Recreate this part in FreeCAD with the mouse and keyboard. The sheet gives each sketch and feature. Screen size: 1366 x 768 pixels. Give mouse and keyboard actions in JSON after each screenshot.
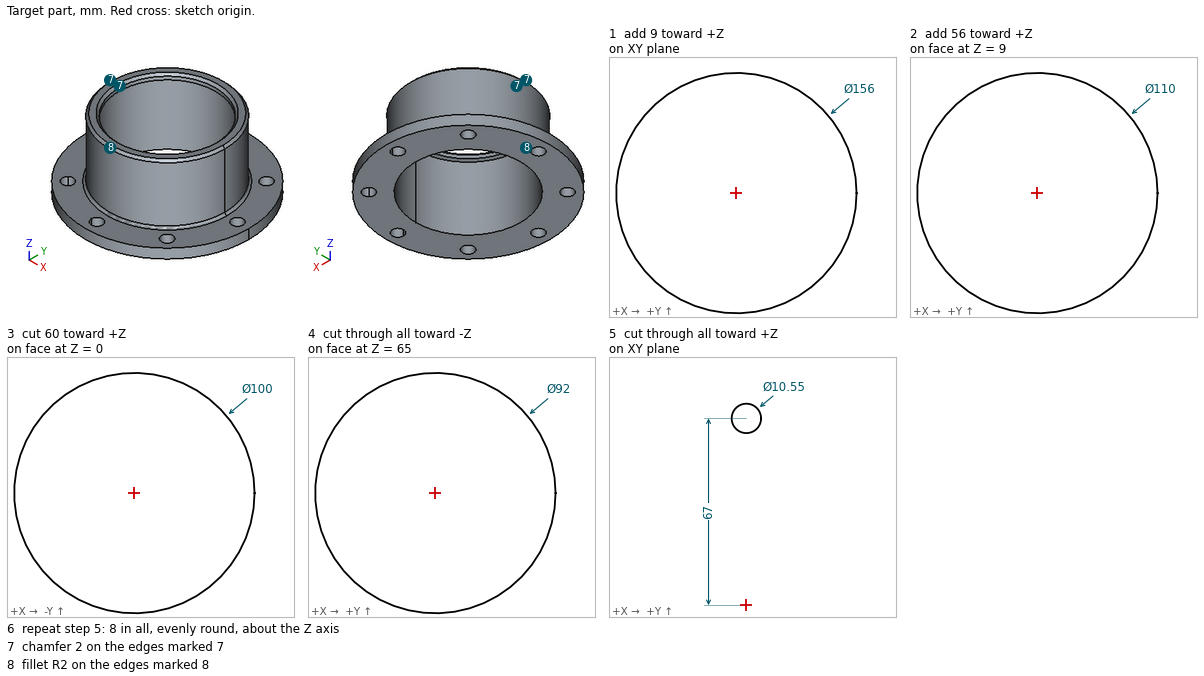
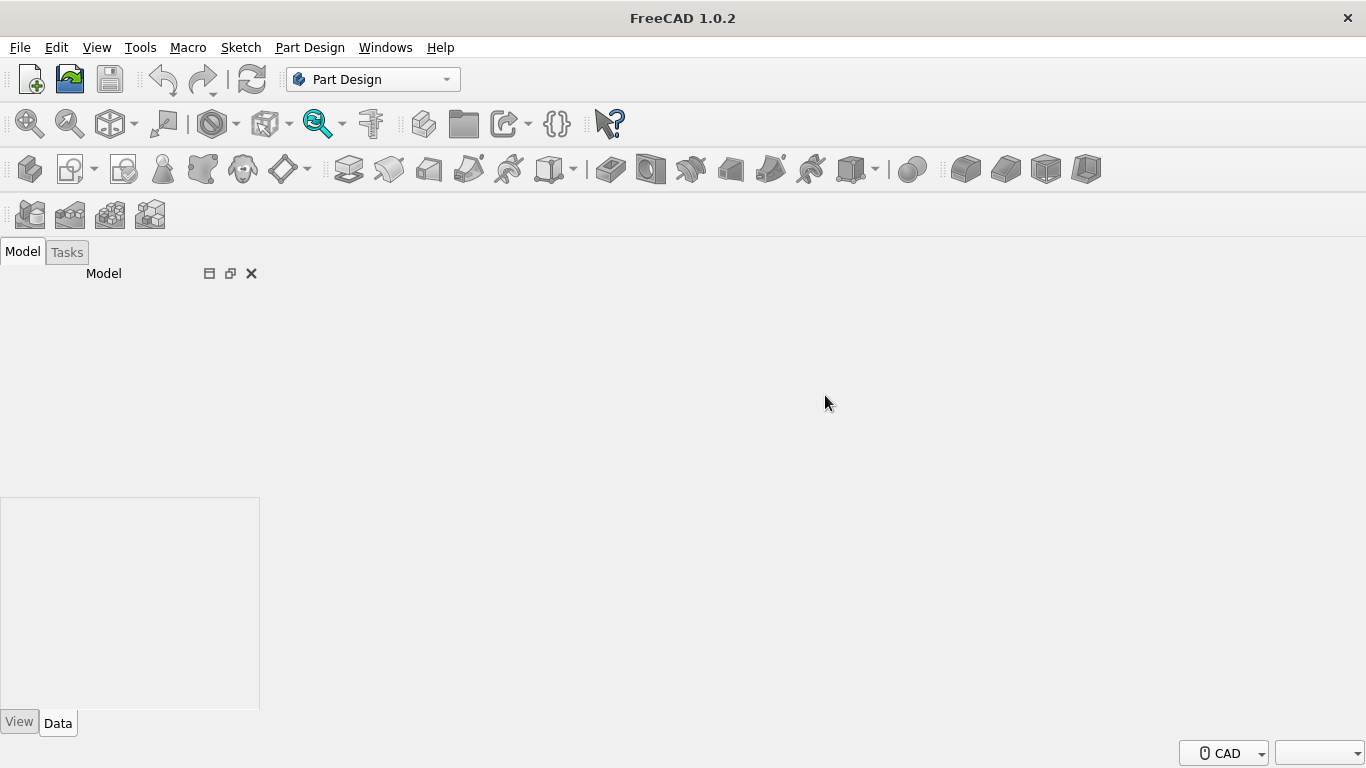
{"action": "key", "text": "ctrl+n"}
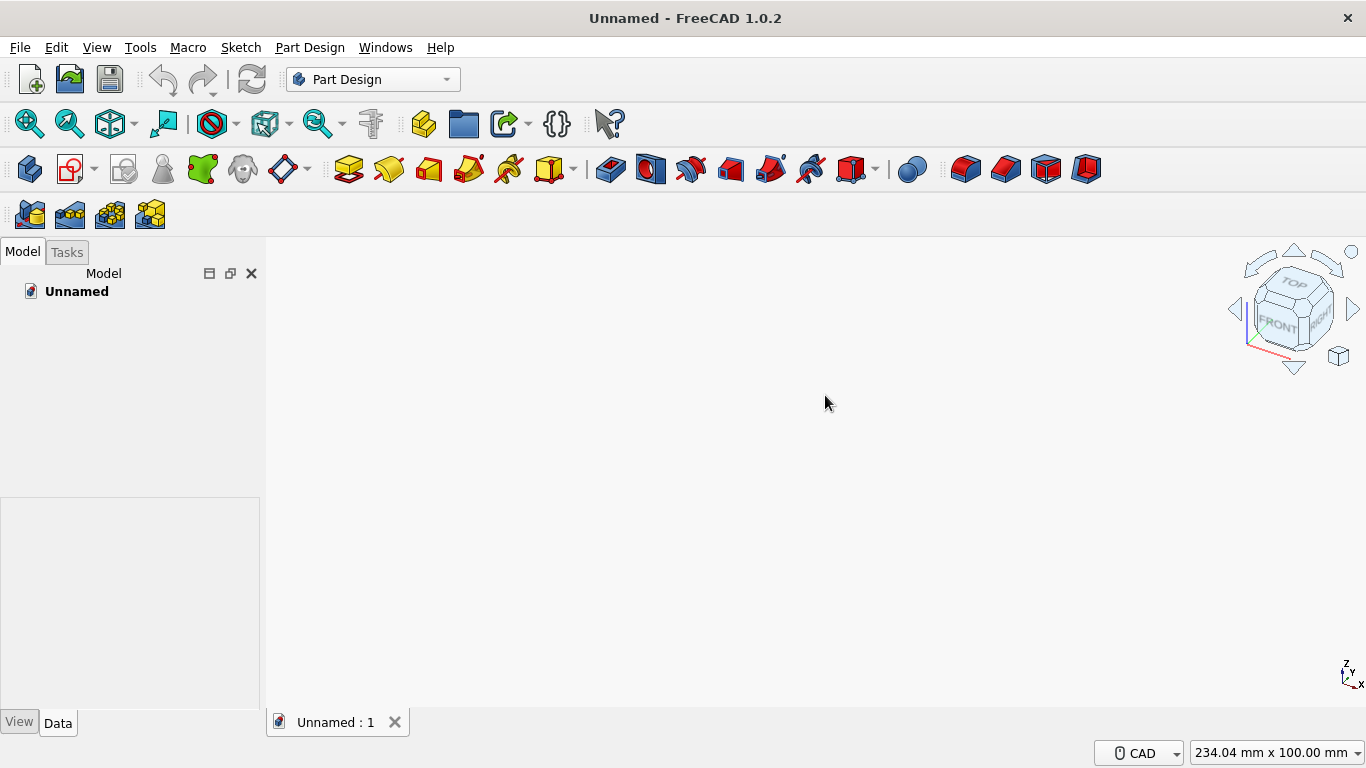
{"action": "left_click", "coordinate": [70, 170]}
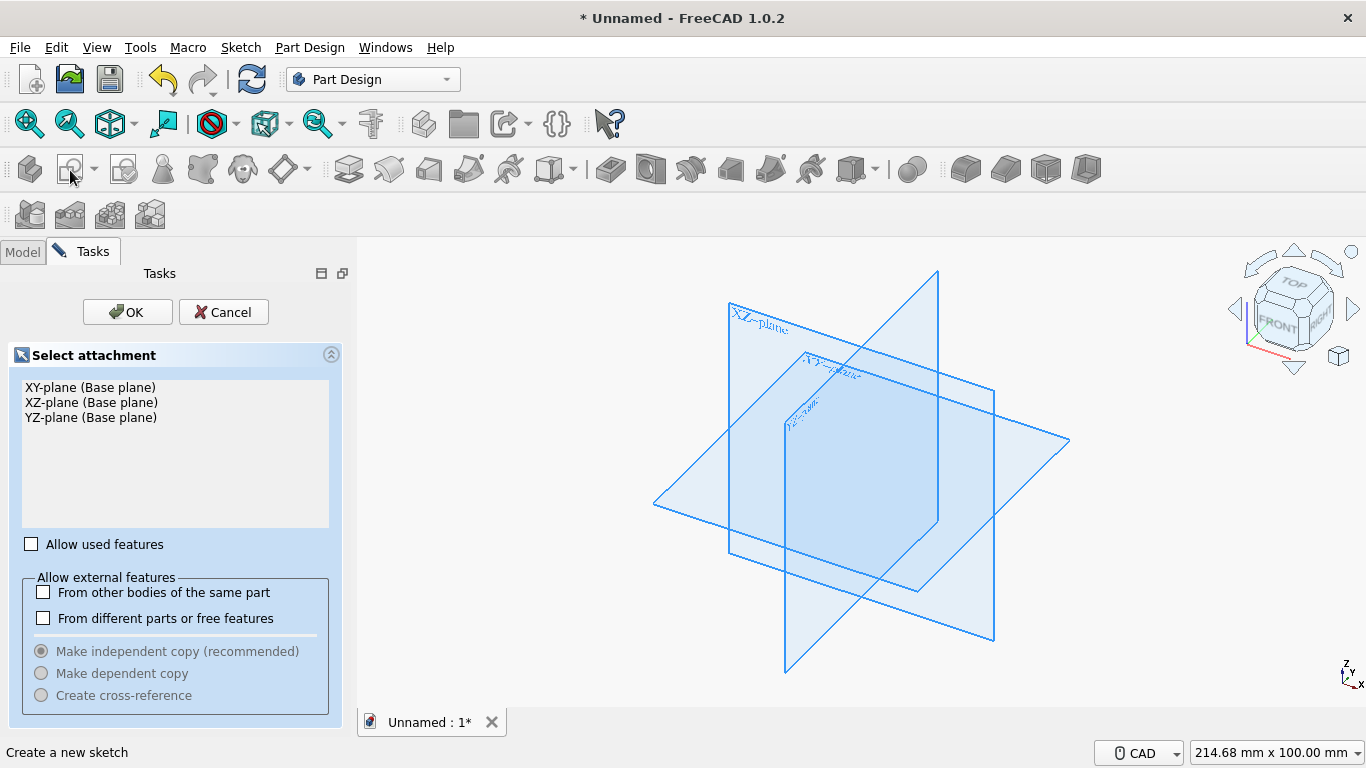
{"action": "left_click", "coordinate": [82, 388]}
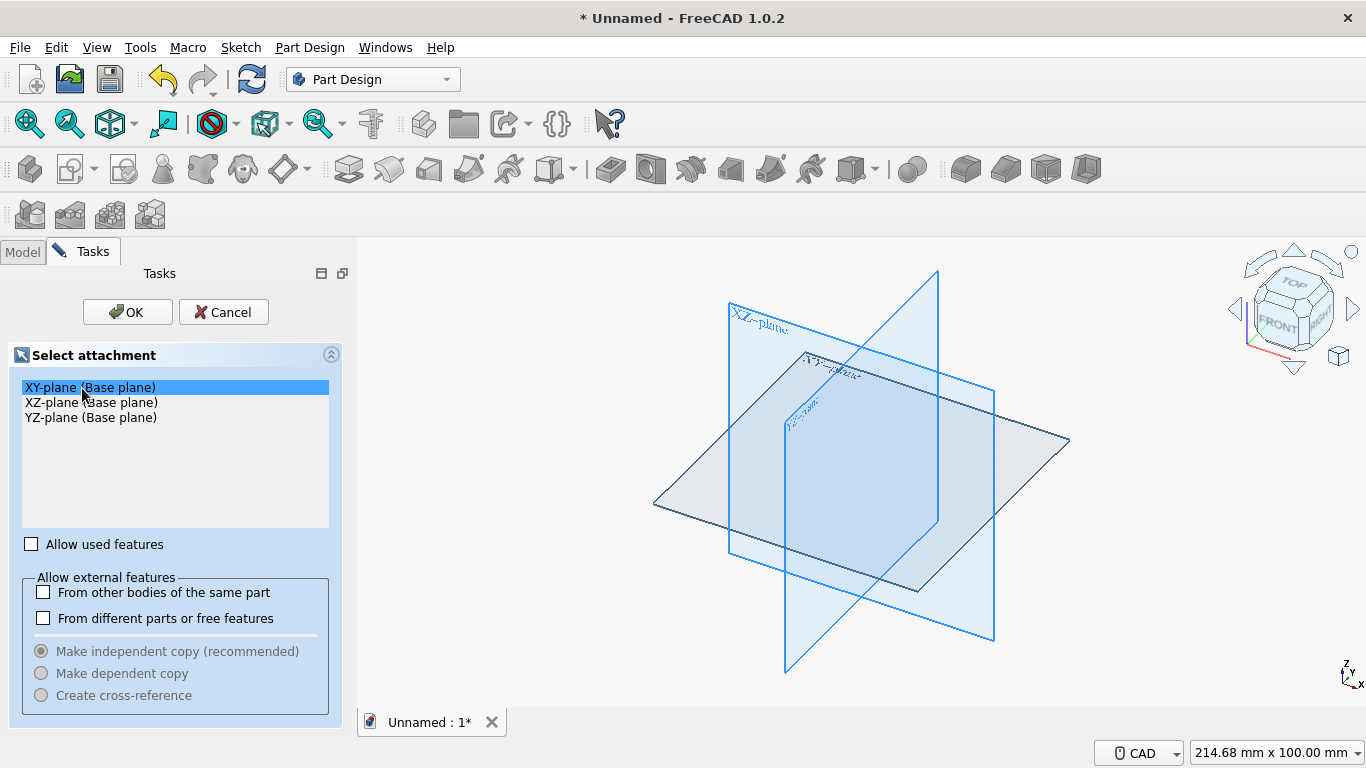
{"action": "left_click", "coordinate": [128, 312]}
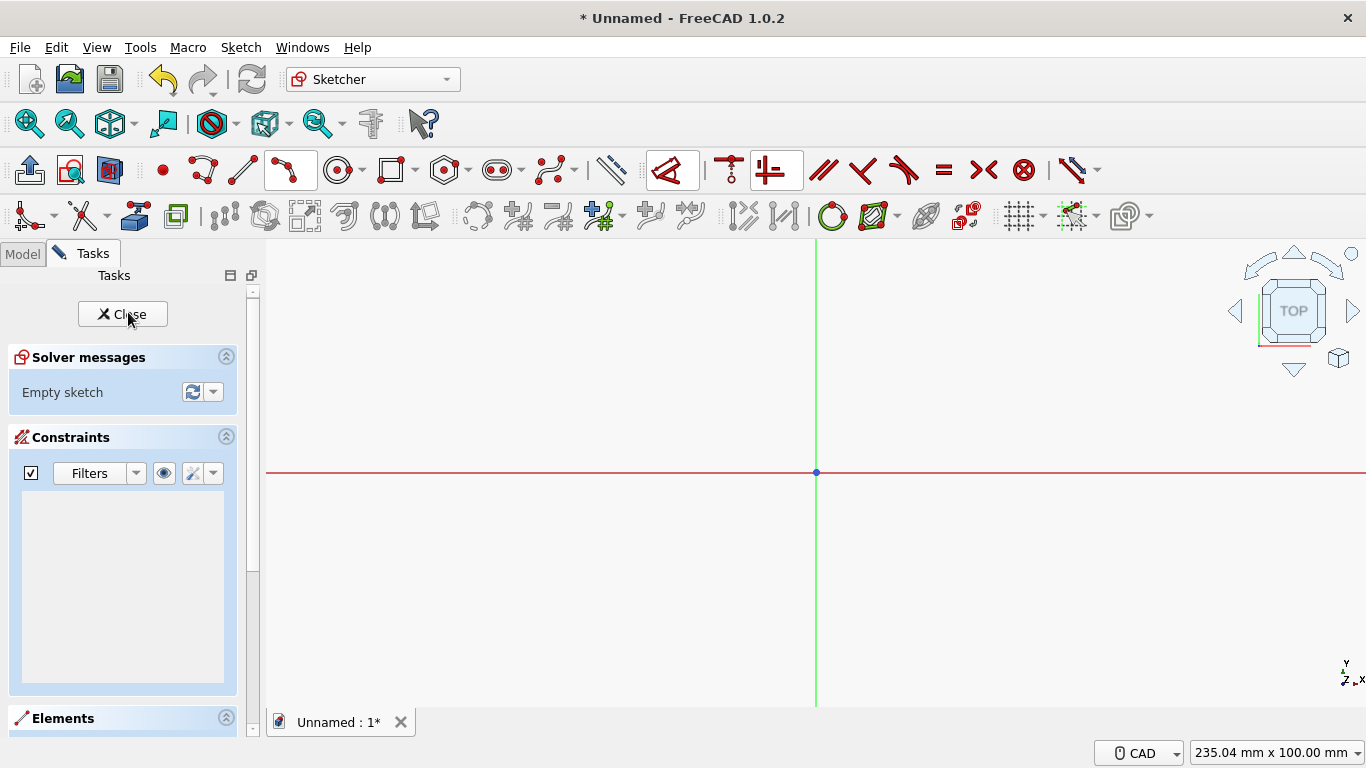
{"action": "scroll", "coordinate": [708, 473], "scroll_direction": "down", "scroll_amount": 5}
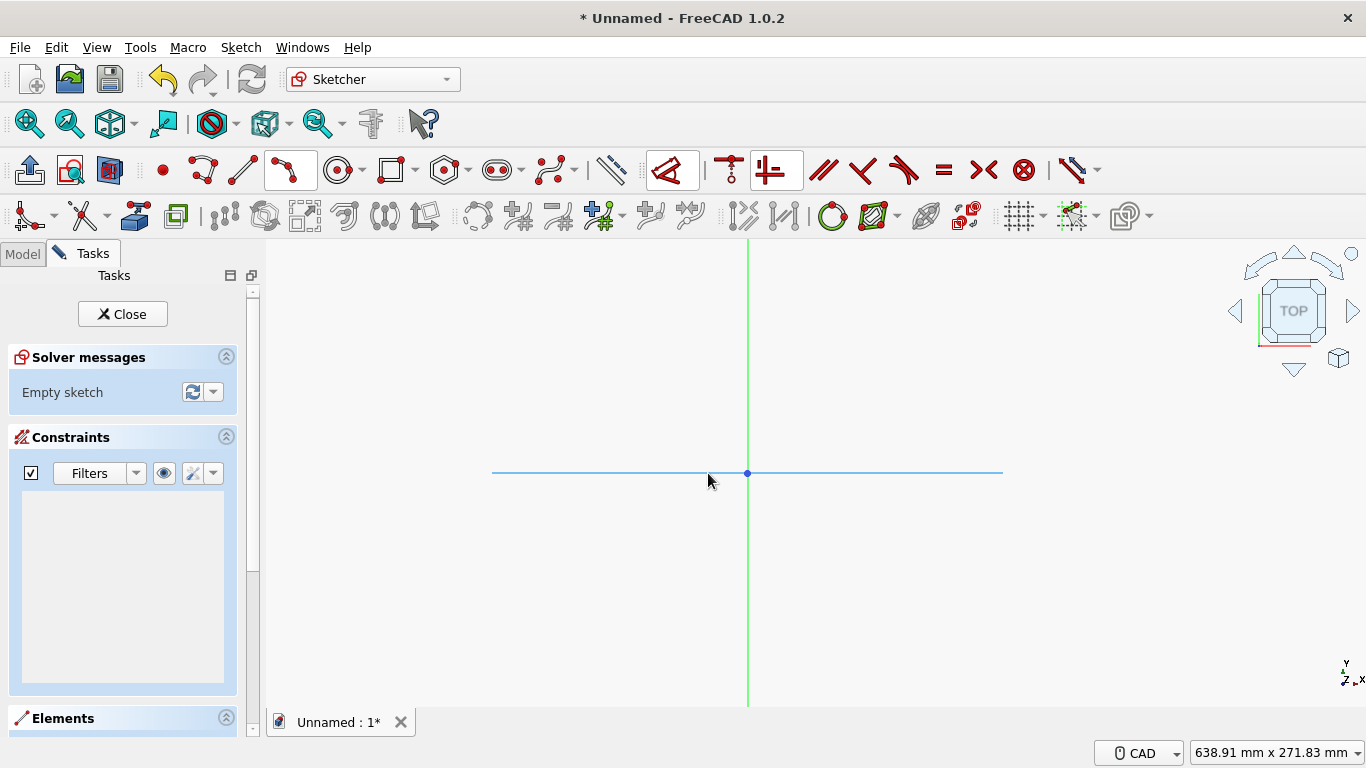
{"action": "left_click", "coordinate": [338, 170]}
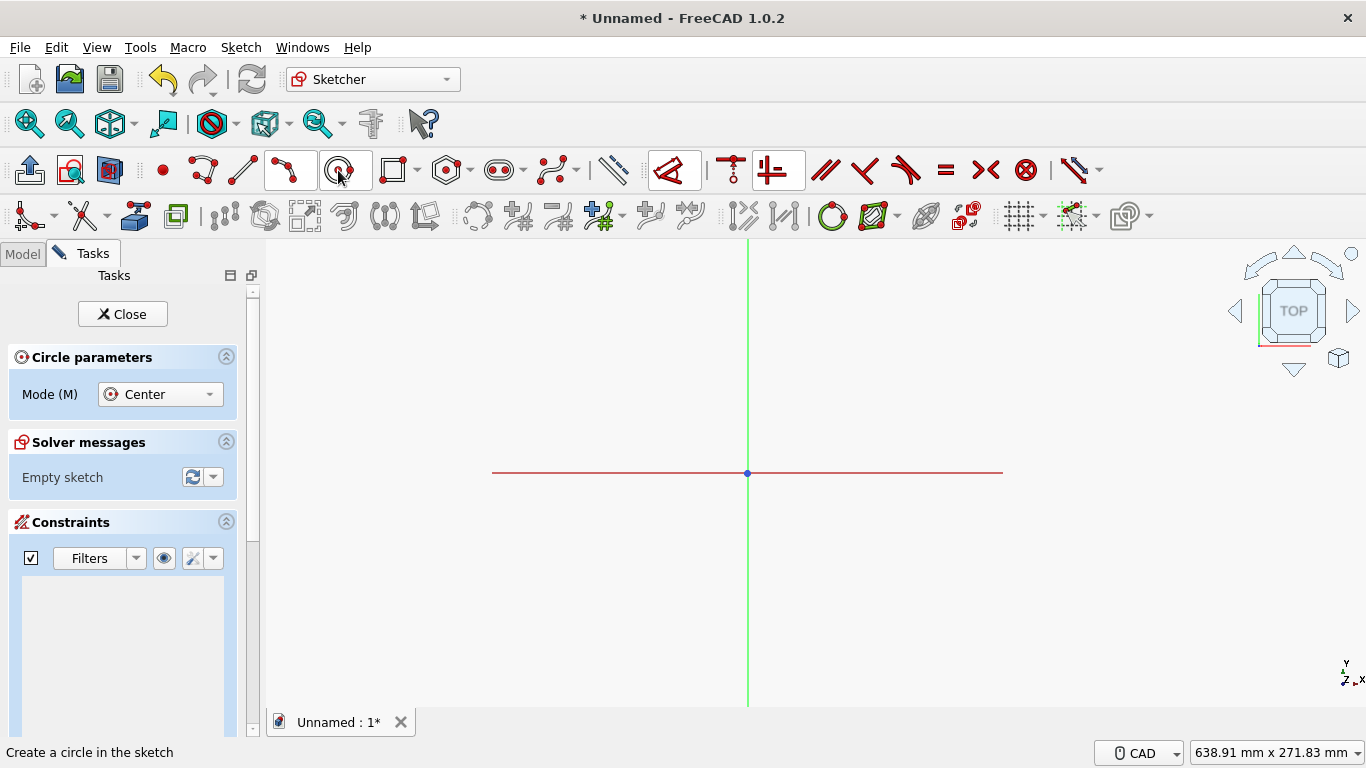
{"action": "left_click", "coordinate": [748, 473]}
{"action": "left_click", "coordinate": [843, 378]}
{"action": "key", "text": "Escape"}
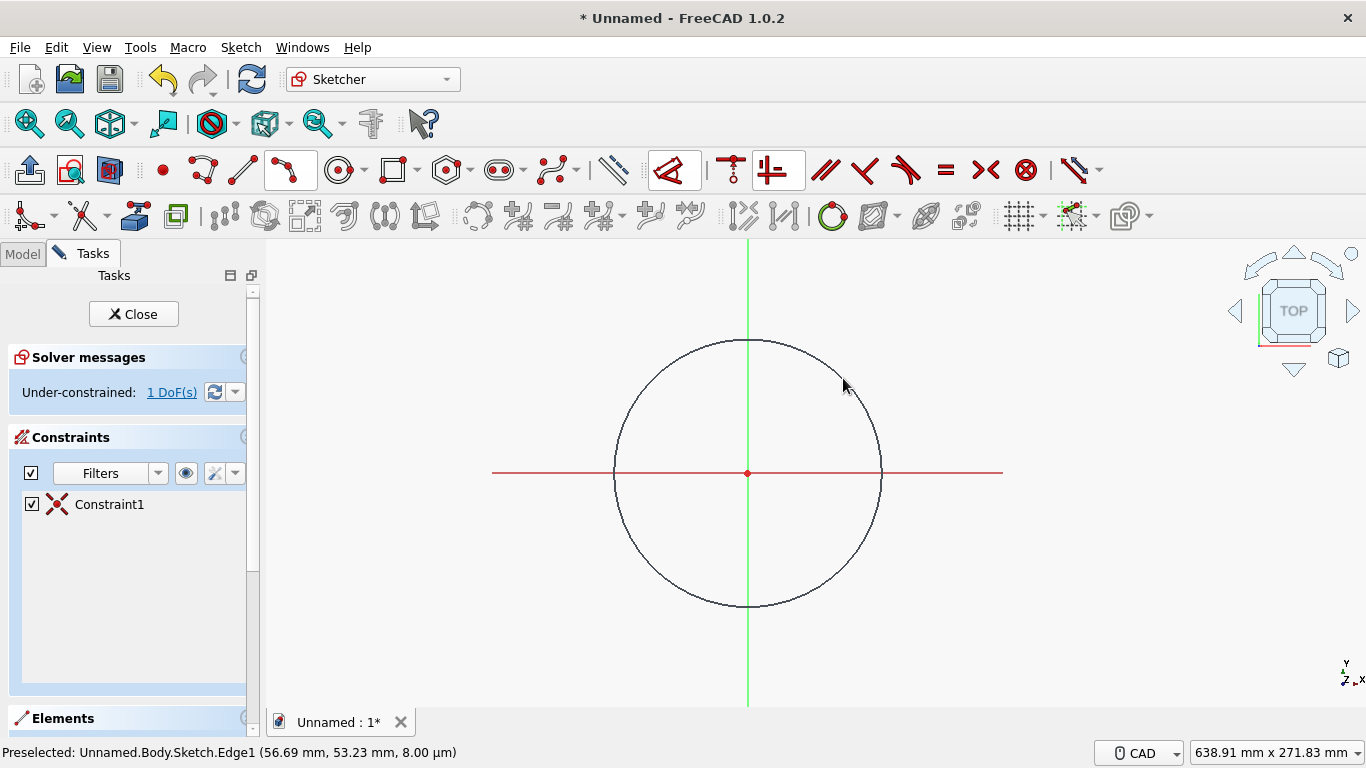
{"action": "left_click", "coordinate": [668, 170]}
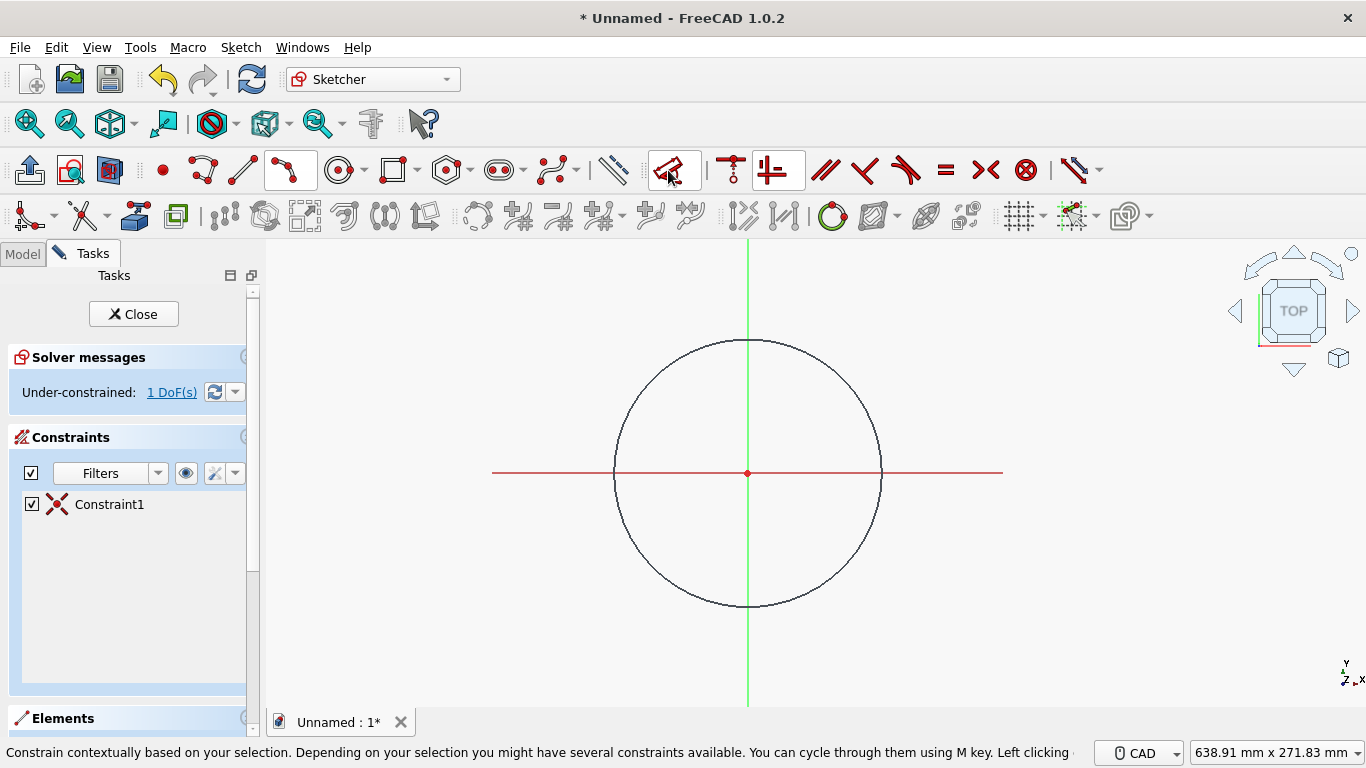
{"action": "left_click", "coordinate": [842, 378]}
{"action": "left_click", "coordinate": [864, 355]}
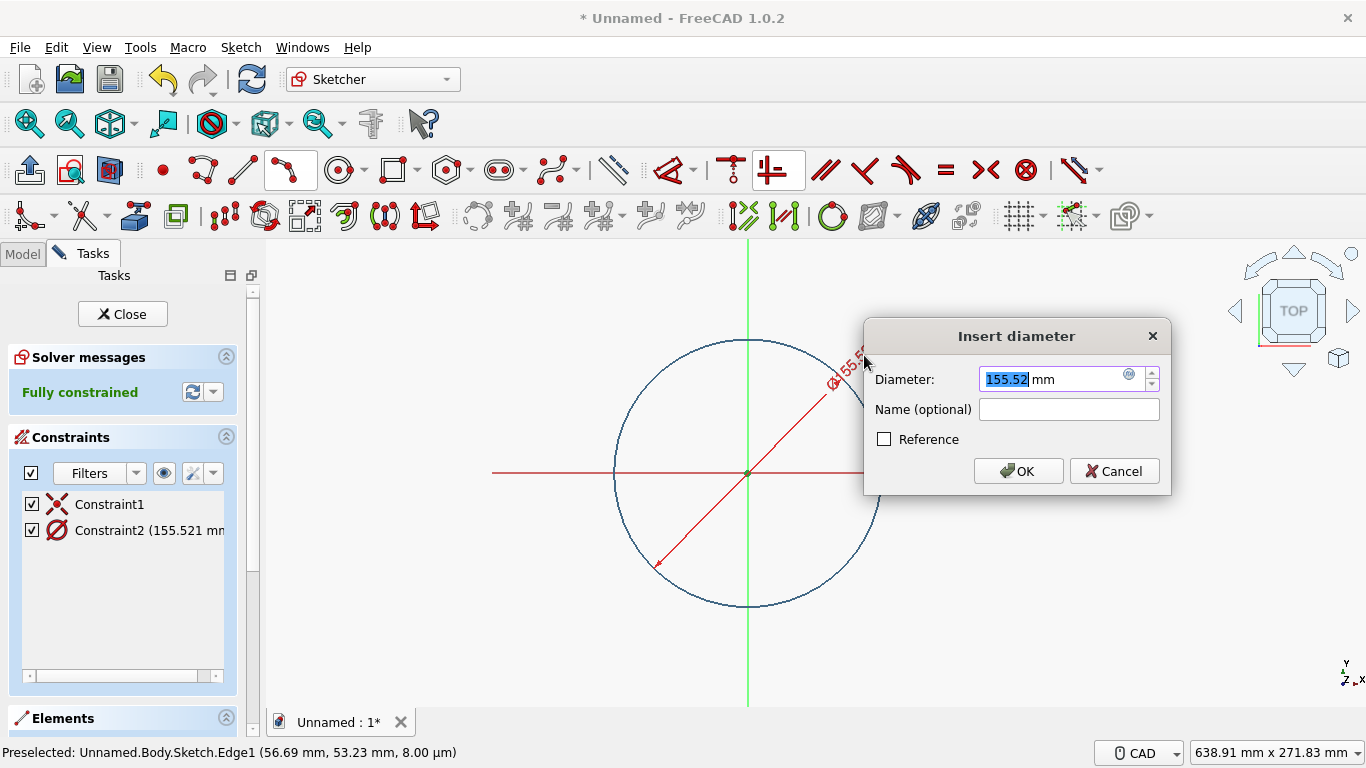
{"action": "type", "text": "156"}
{"action": "key", "text": "Return"}
{"action": "key", "text": "Escape"}